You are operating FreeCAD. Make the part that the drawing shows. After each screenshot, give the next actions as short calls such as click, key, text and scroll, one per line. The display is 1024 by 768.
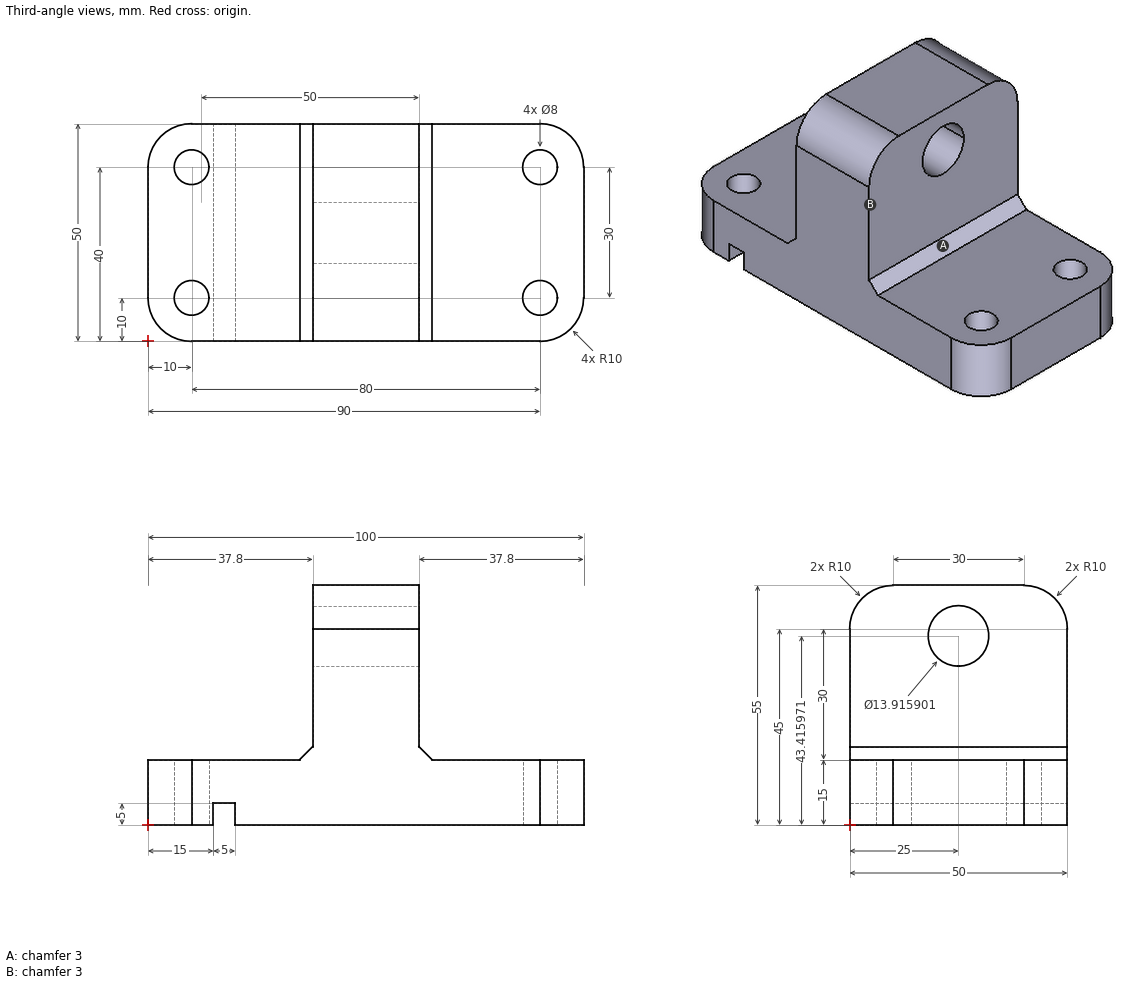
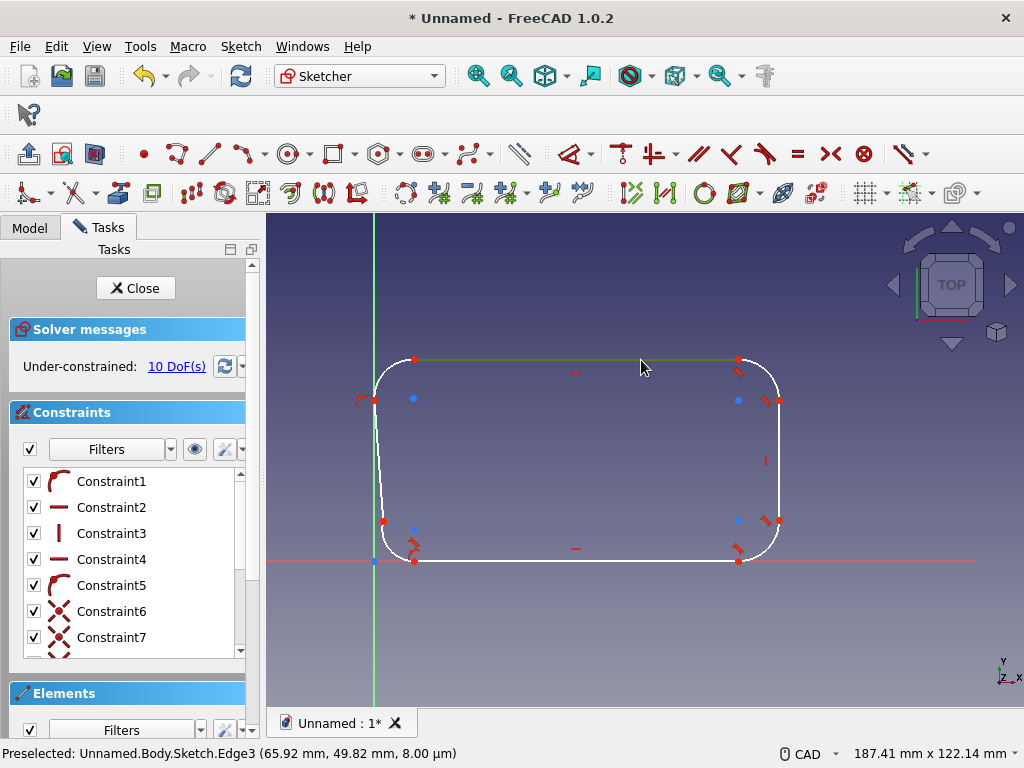
click(396, 364)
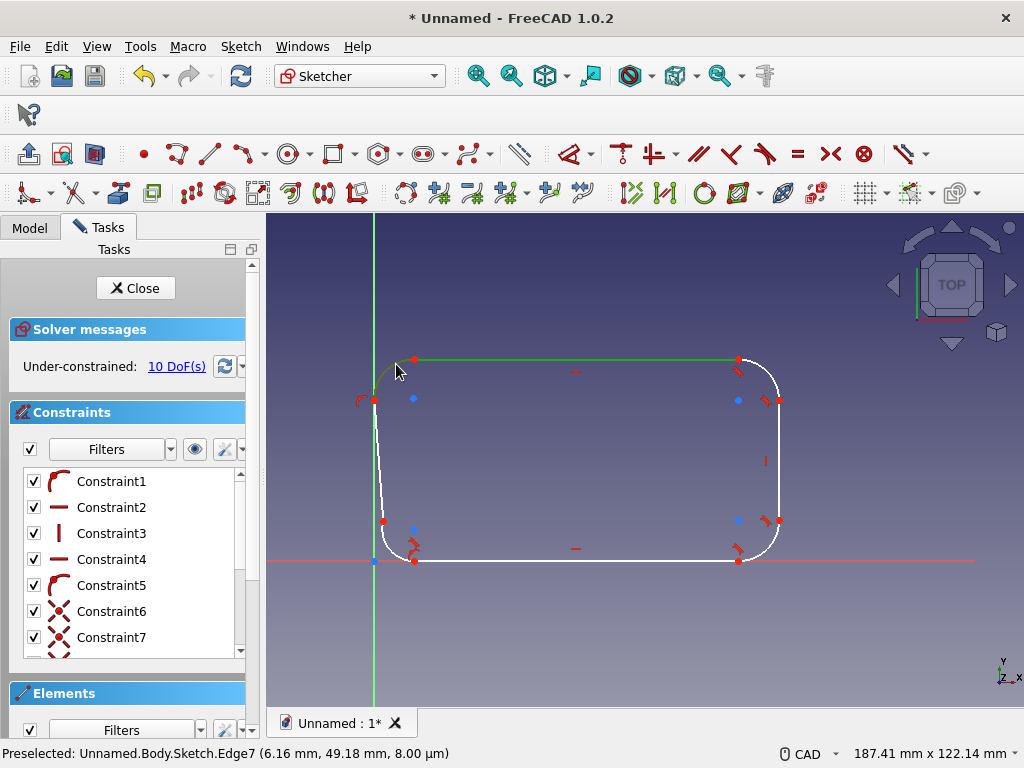
click(765, 154)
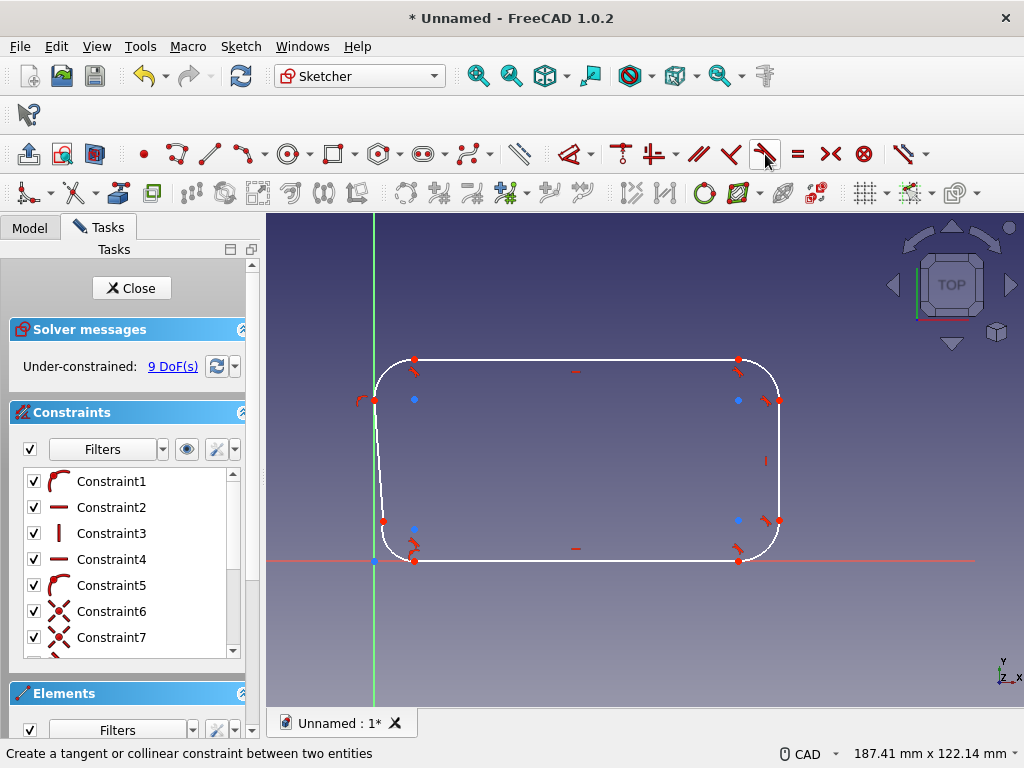
click(377, 437)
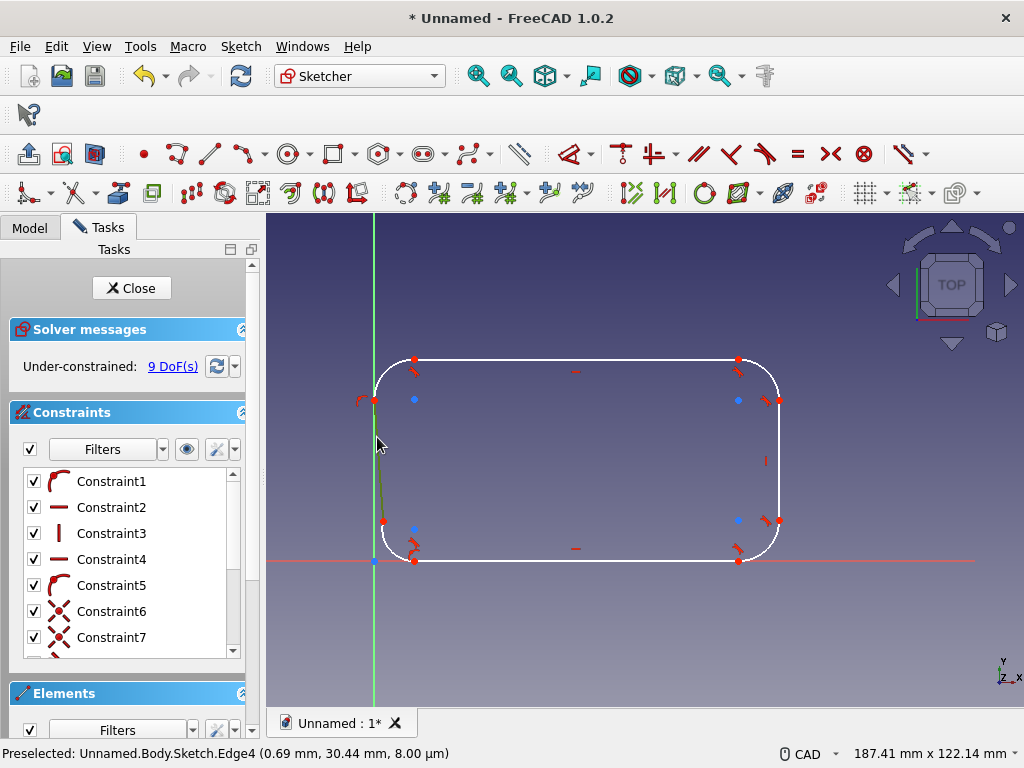
click(396, 364)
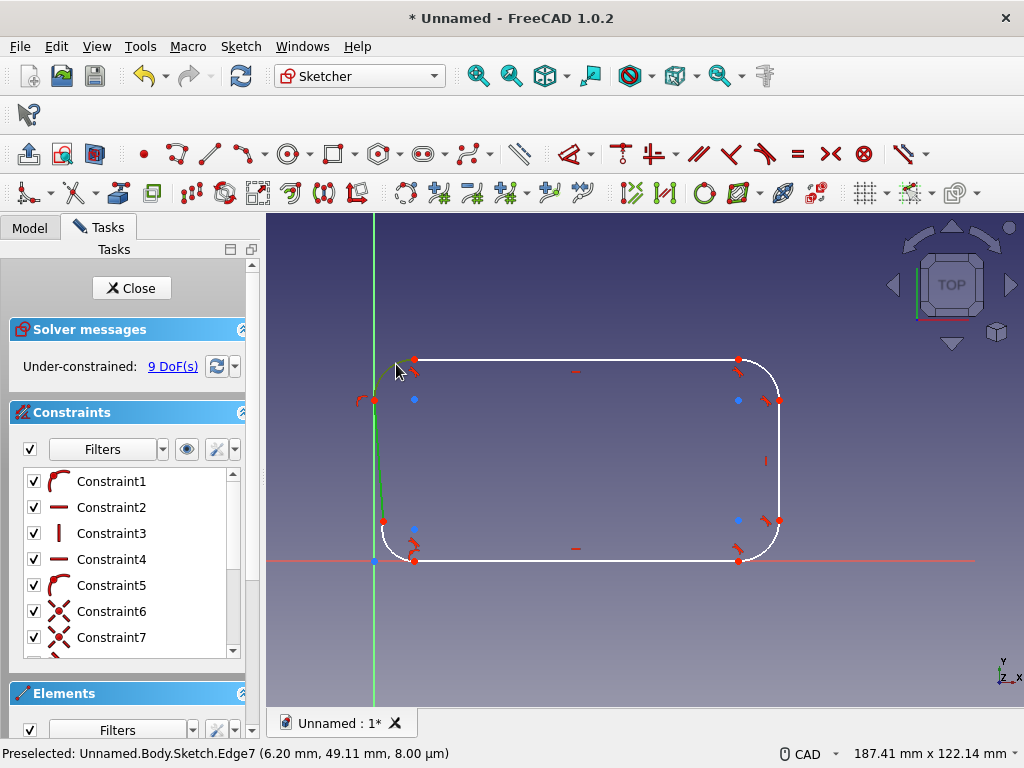
click(765, 154)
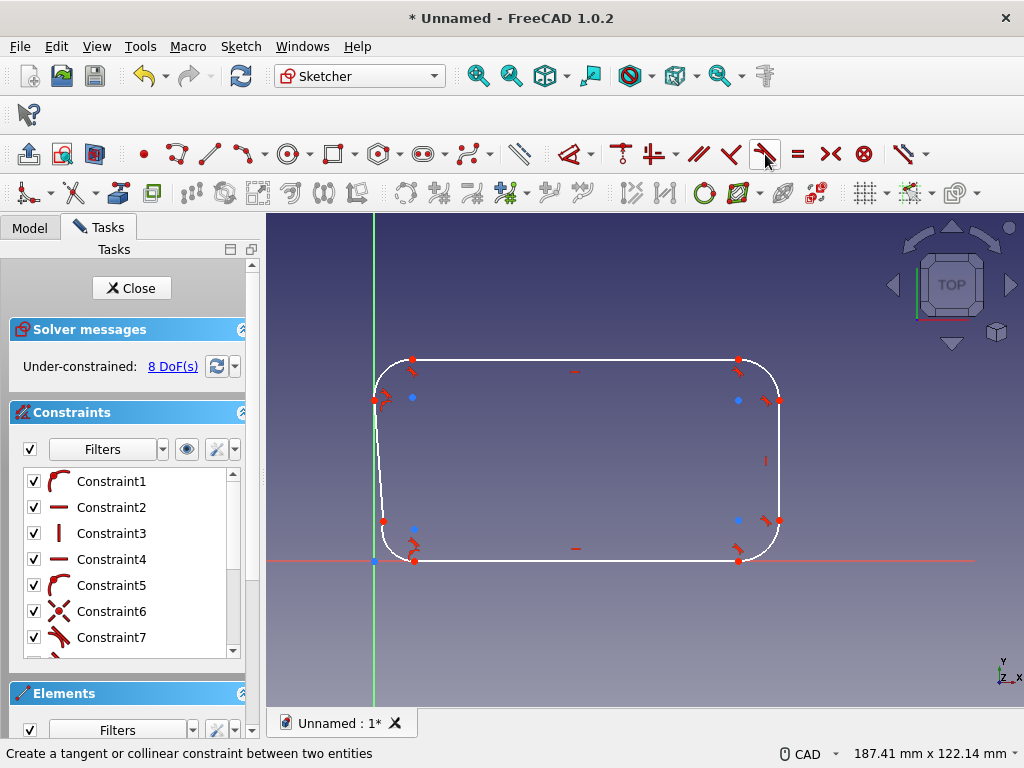
click(377, 437)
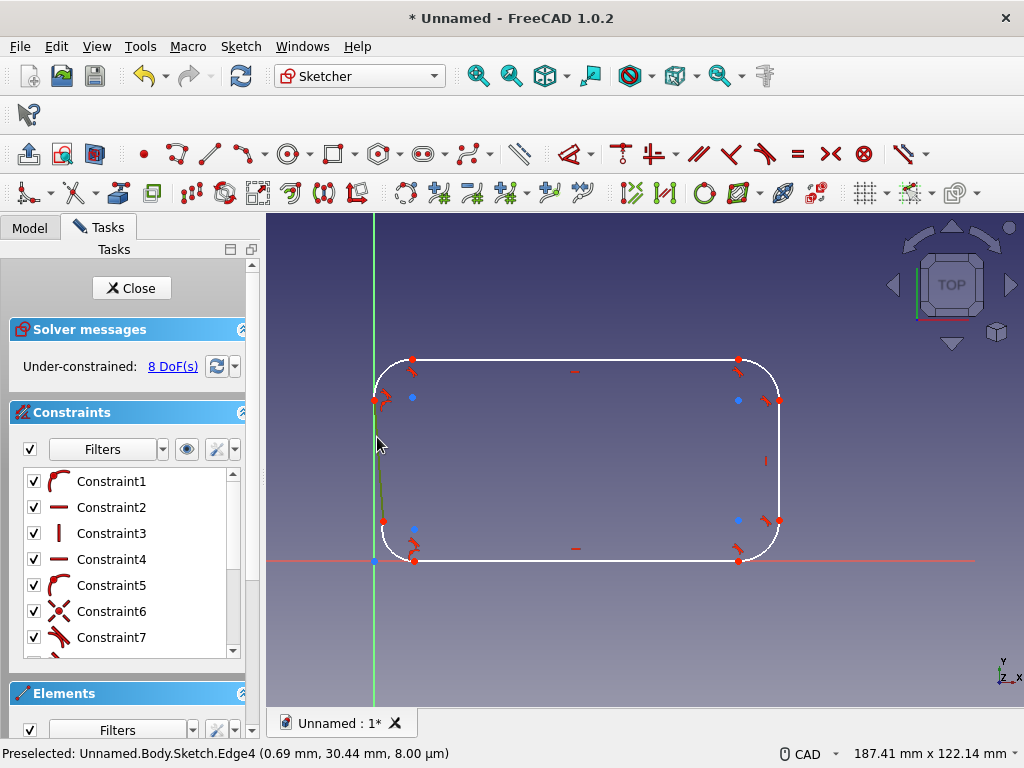
scroll(384, 539, up, 2)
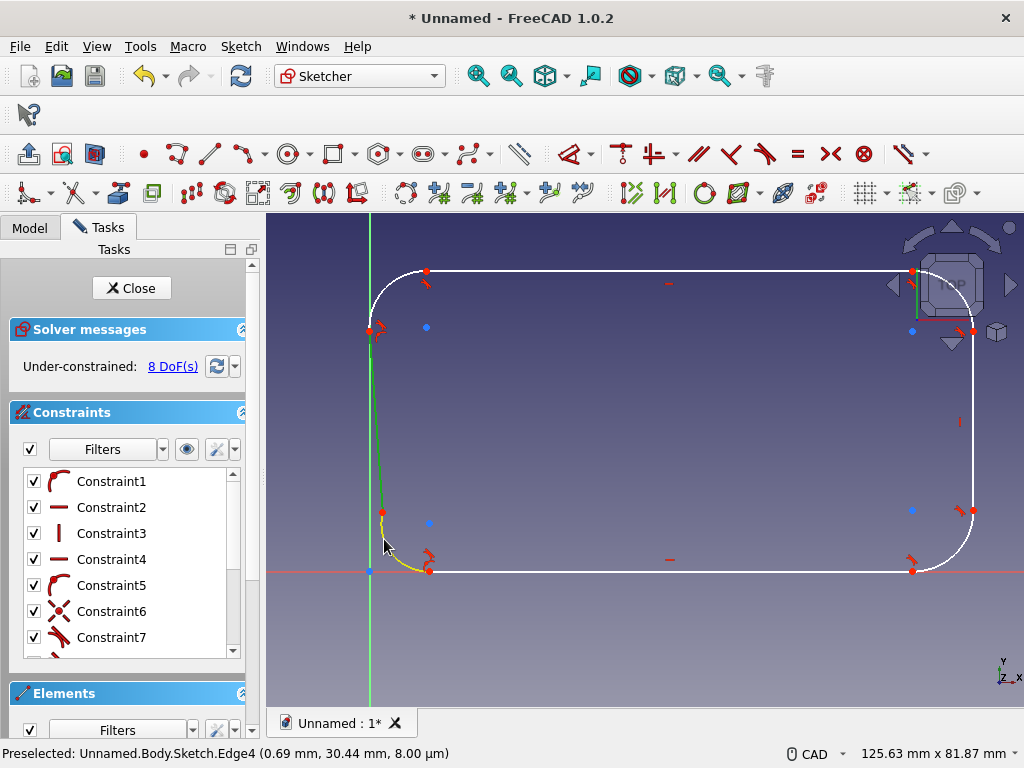
click(384, 538)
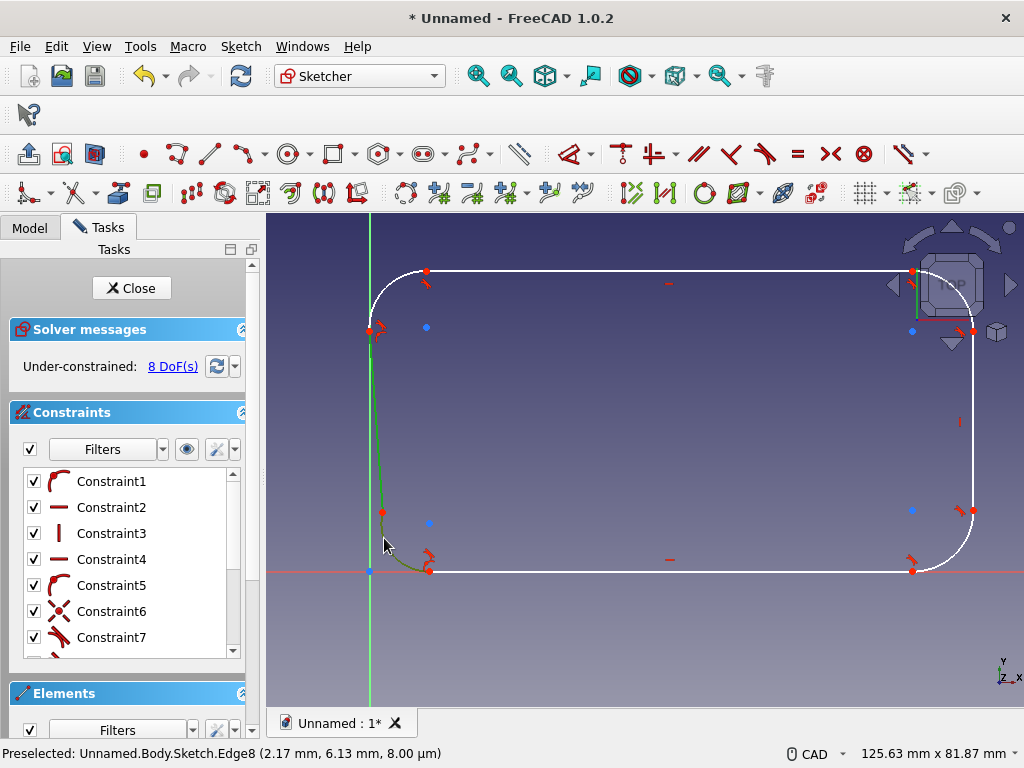
click(765, 154)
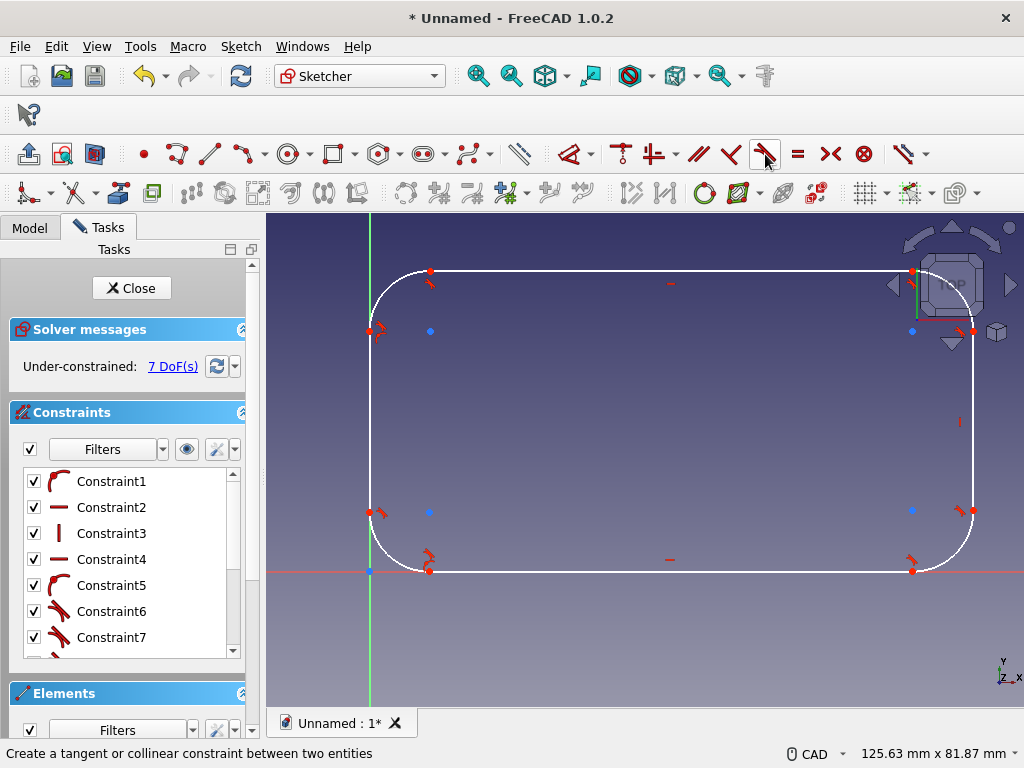
click(370, 386)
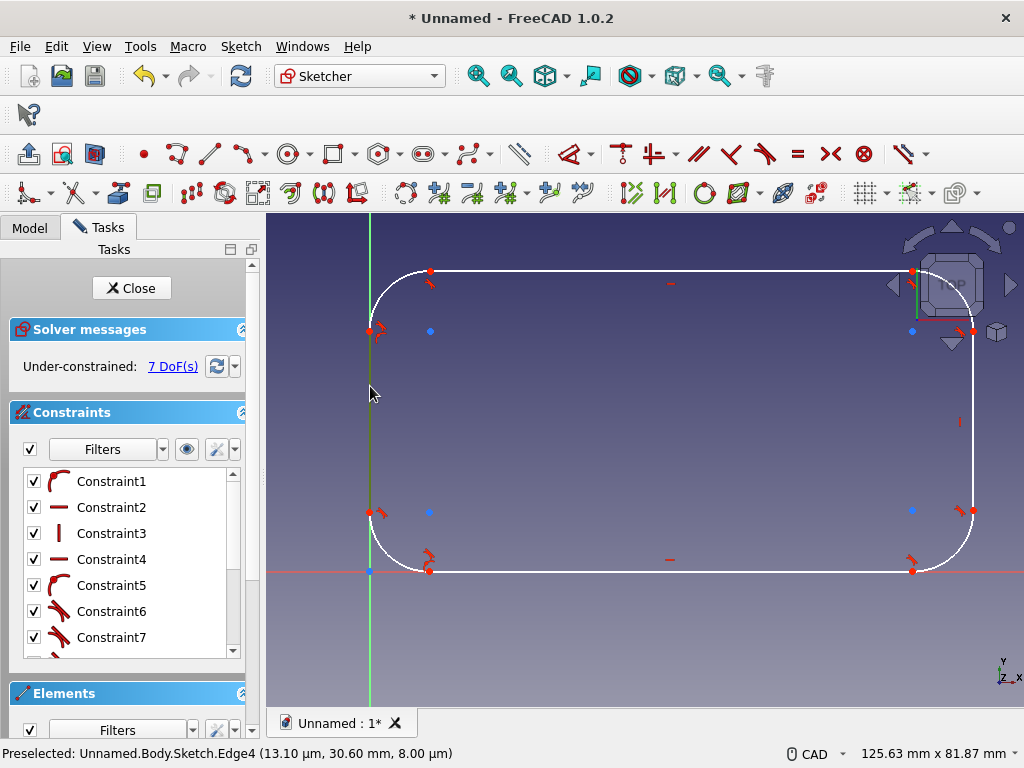
click(676, 154)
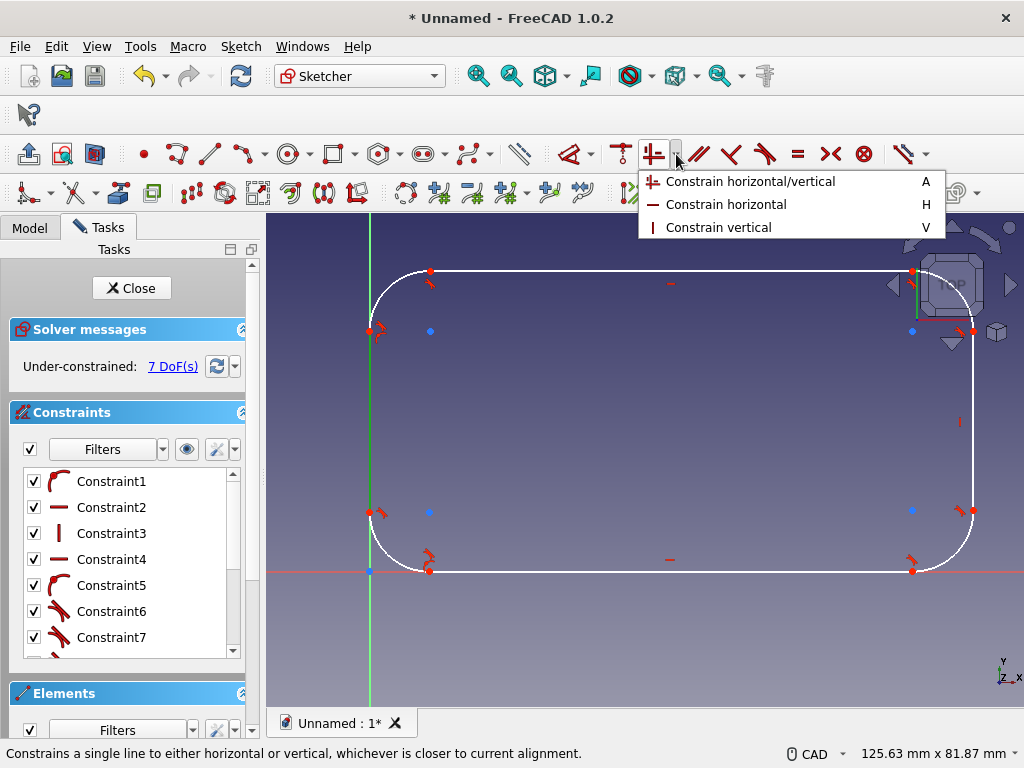
click(792, 228)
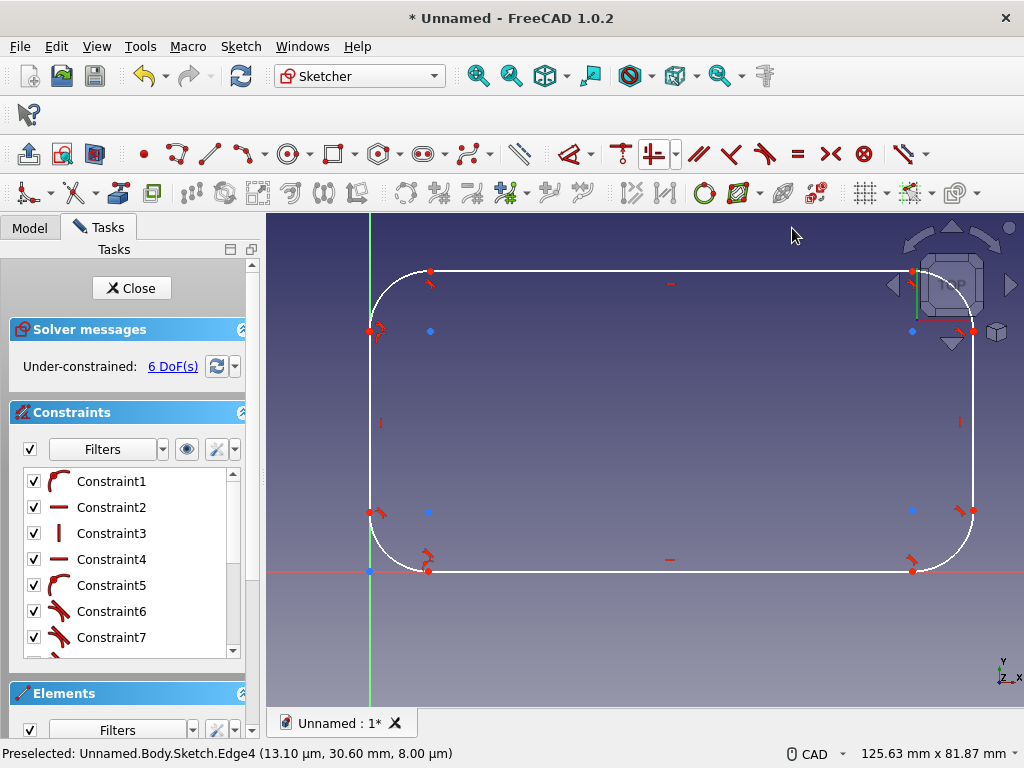
scroll(384, 540, down, 2)